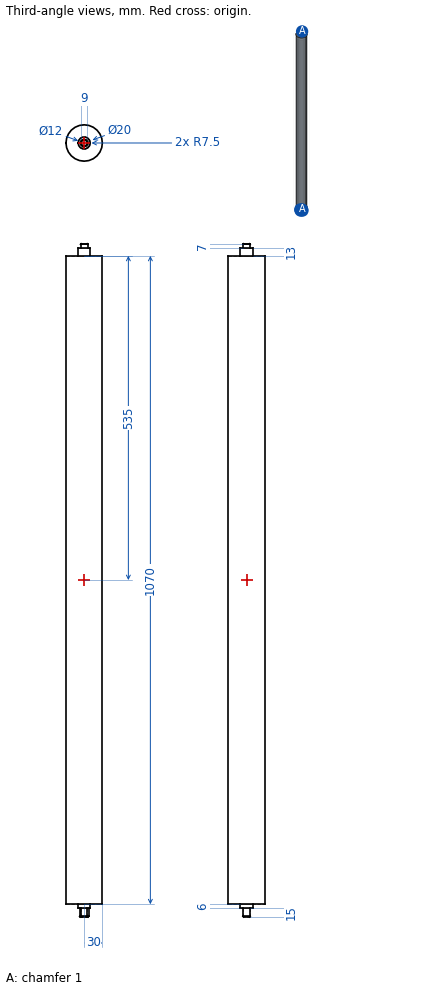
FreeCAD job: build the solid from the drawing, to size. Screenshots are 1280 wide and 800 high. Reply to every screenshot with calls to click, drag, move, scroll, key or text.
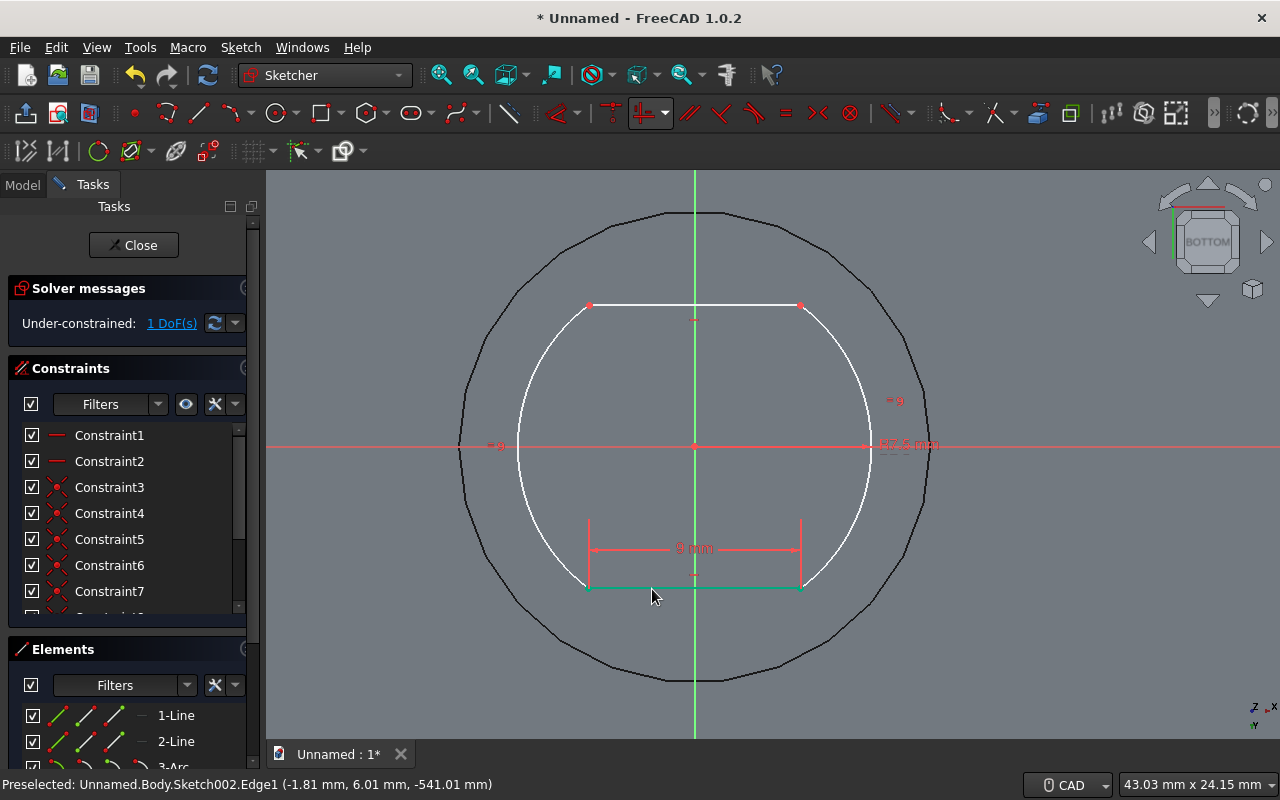
click(737, 305)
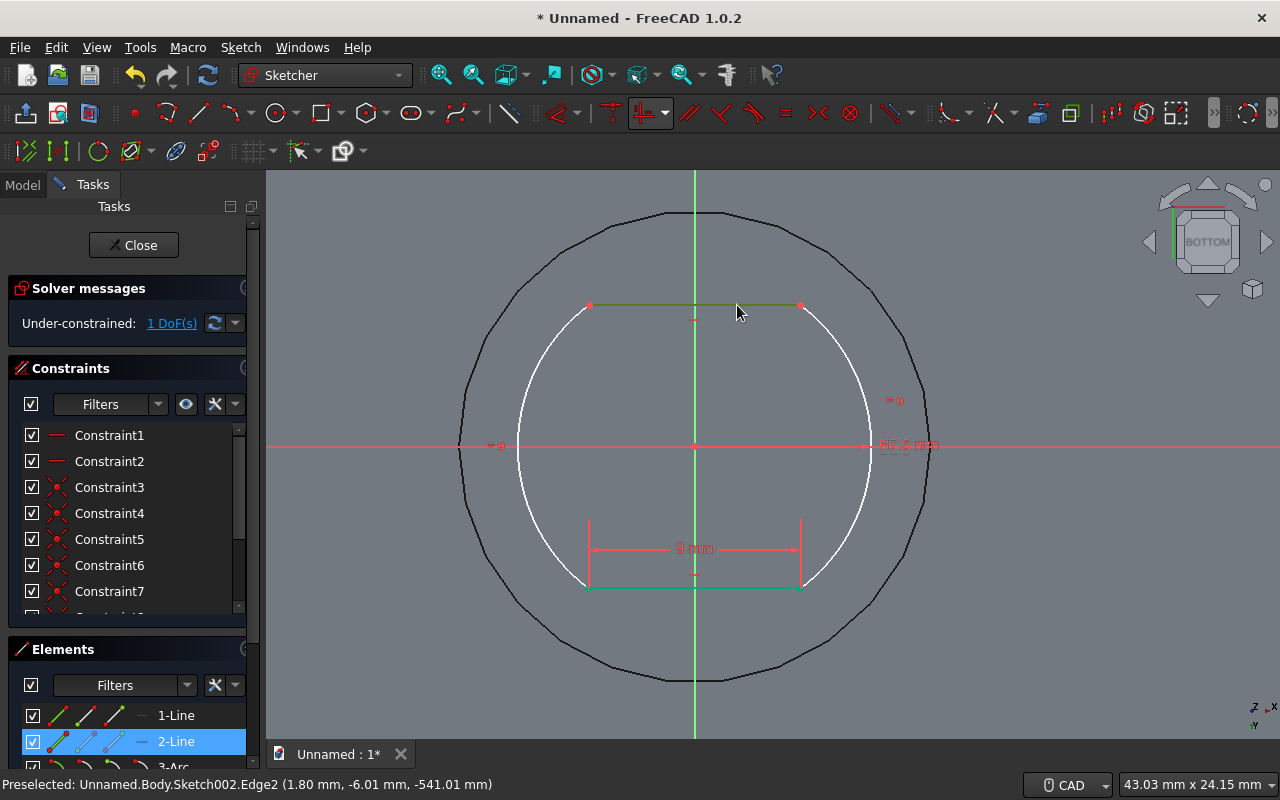
key(l)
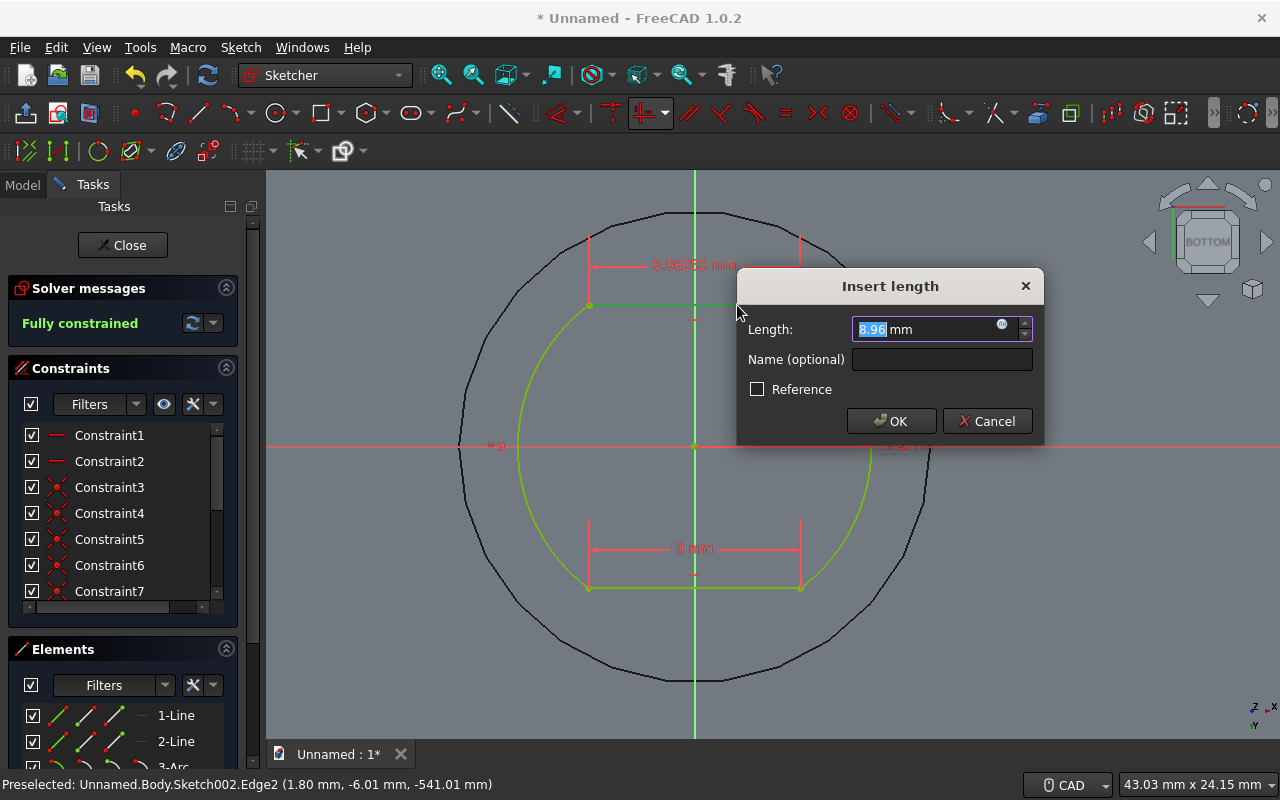
text(9)
key(Return)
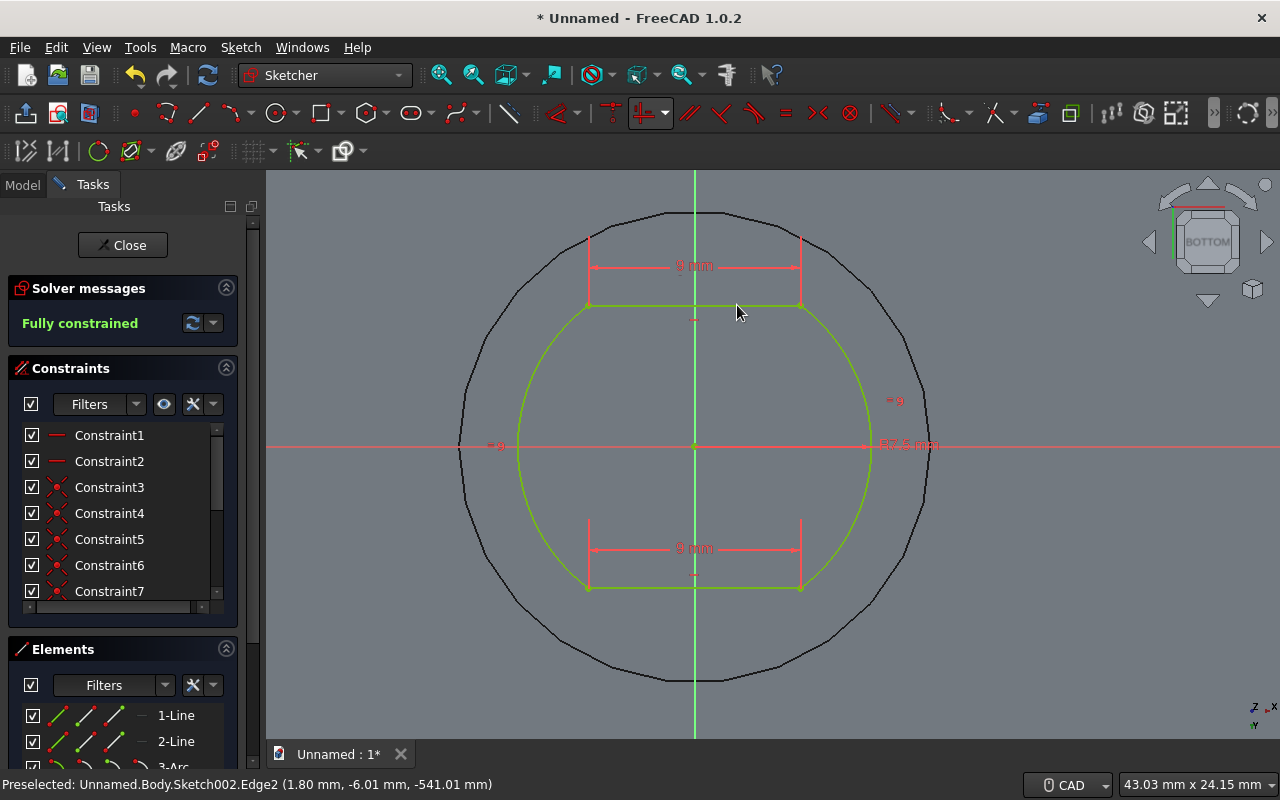
click(123, 245)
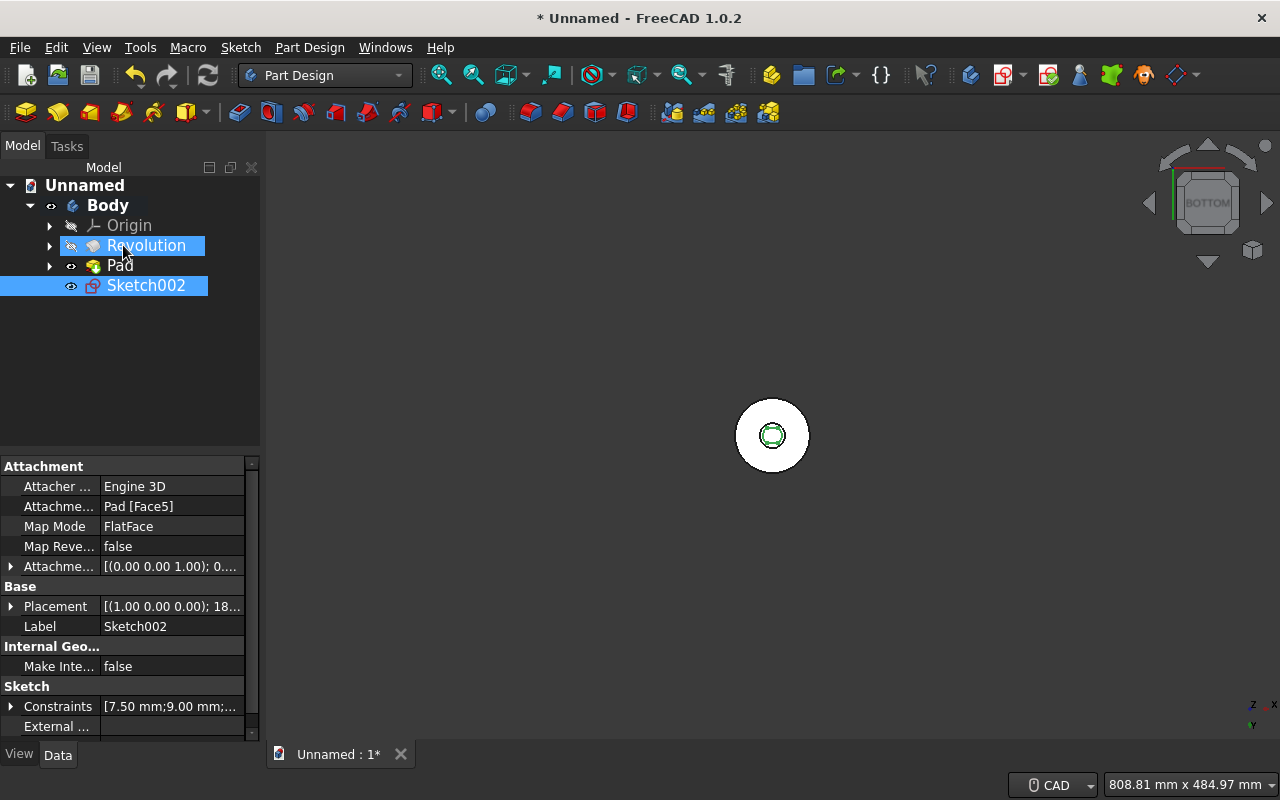
click(26, 112)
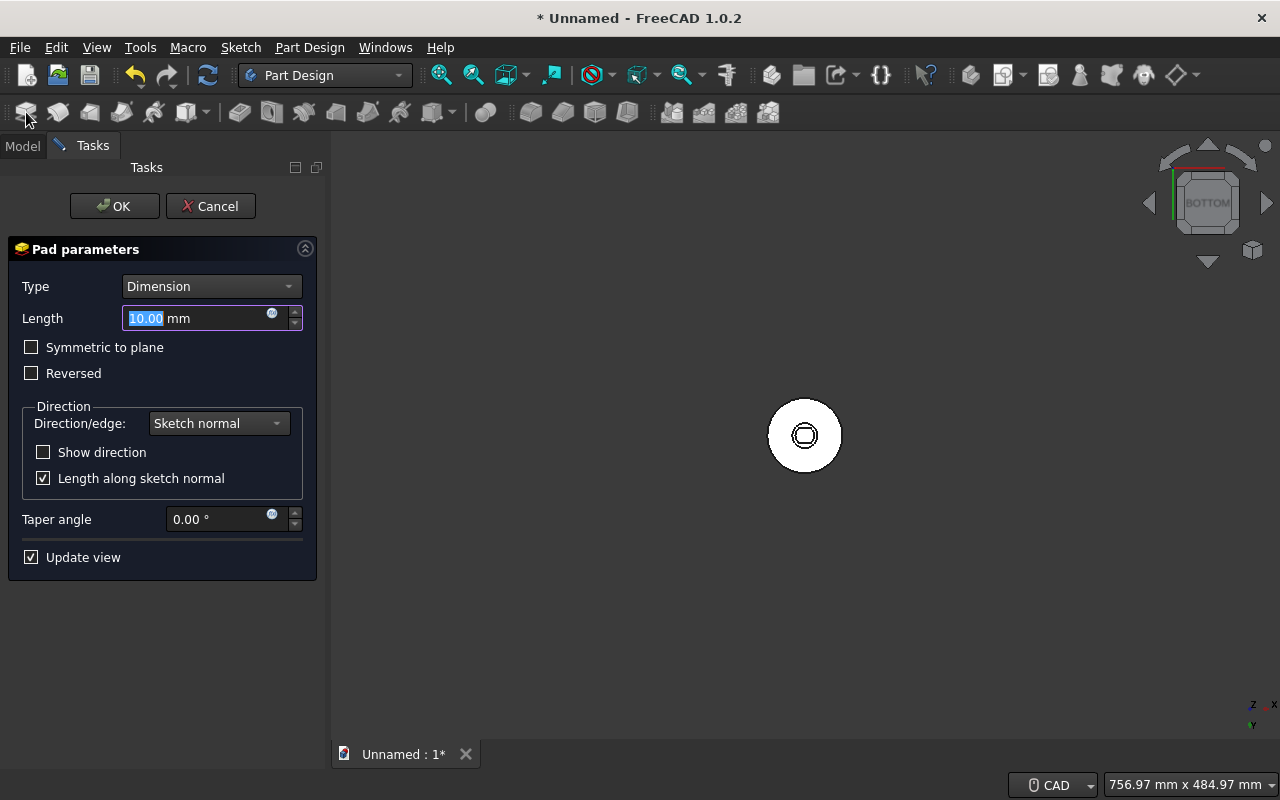
text(15)
key(Tab)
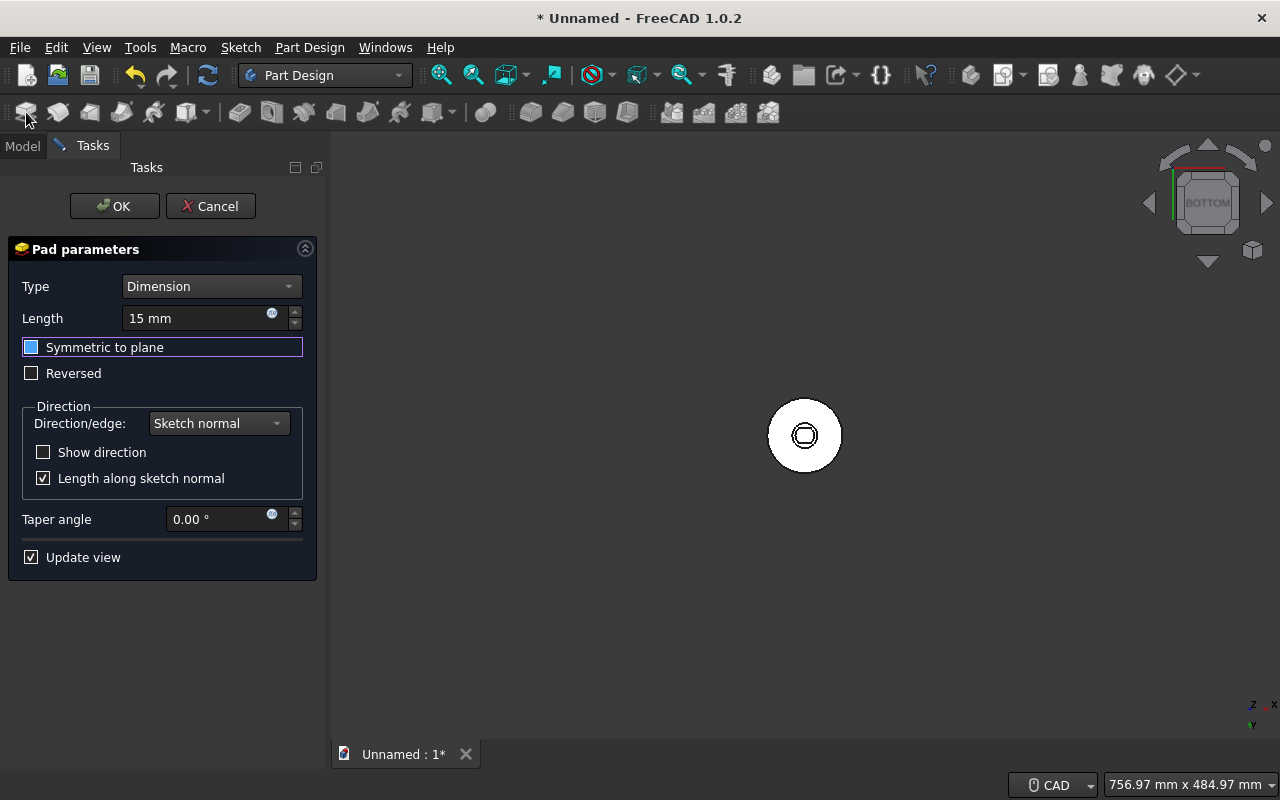
click(115, 206)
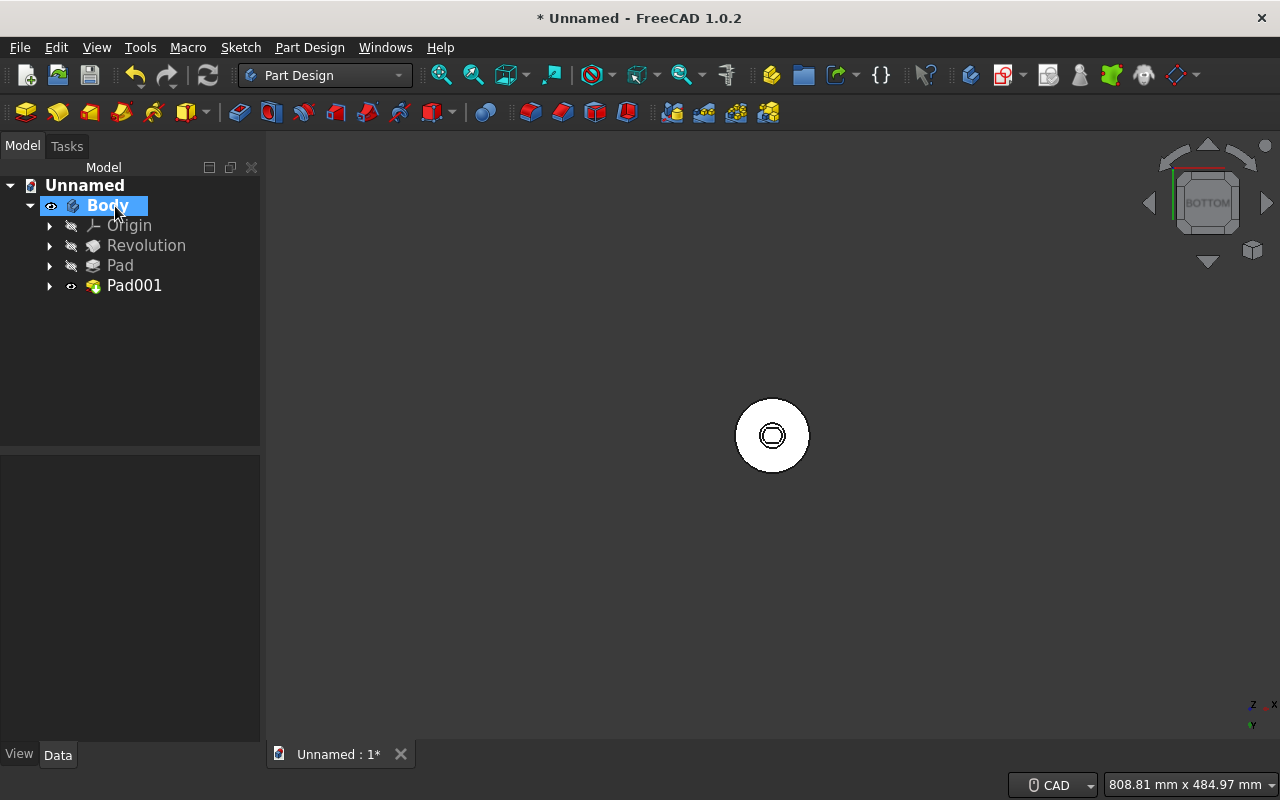
click(442, 76)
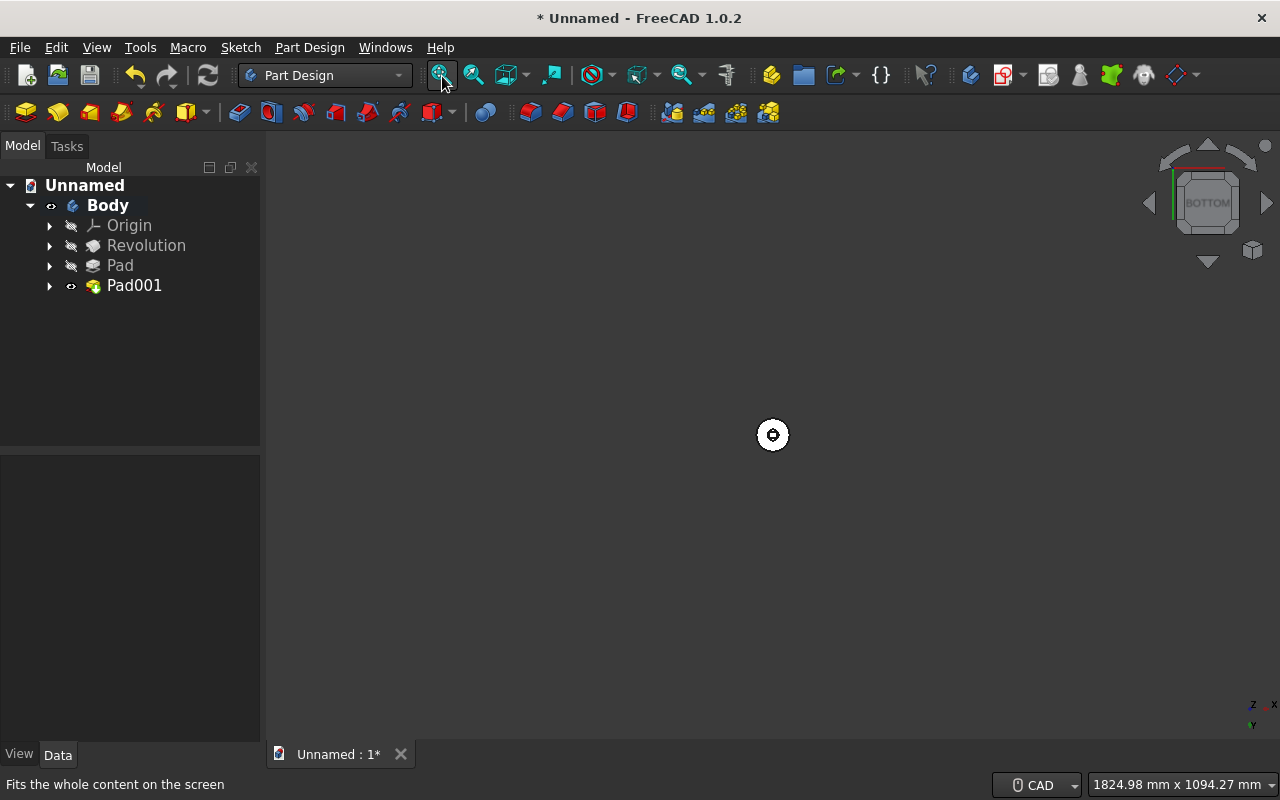
click(50, 226)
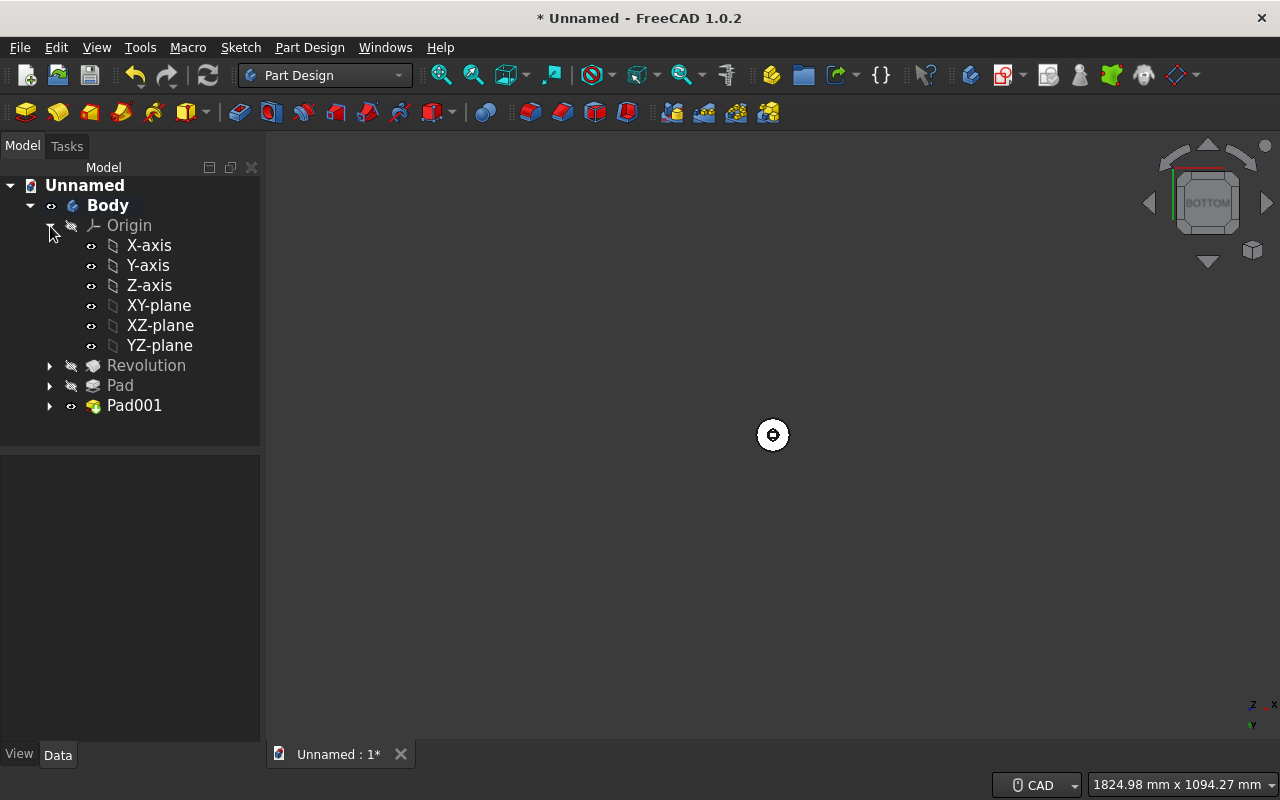
click(136, 306)